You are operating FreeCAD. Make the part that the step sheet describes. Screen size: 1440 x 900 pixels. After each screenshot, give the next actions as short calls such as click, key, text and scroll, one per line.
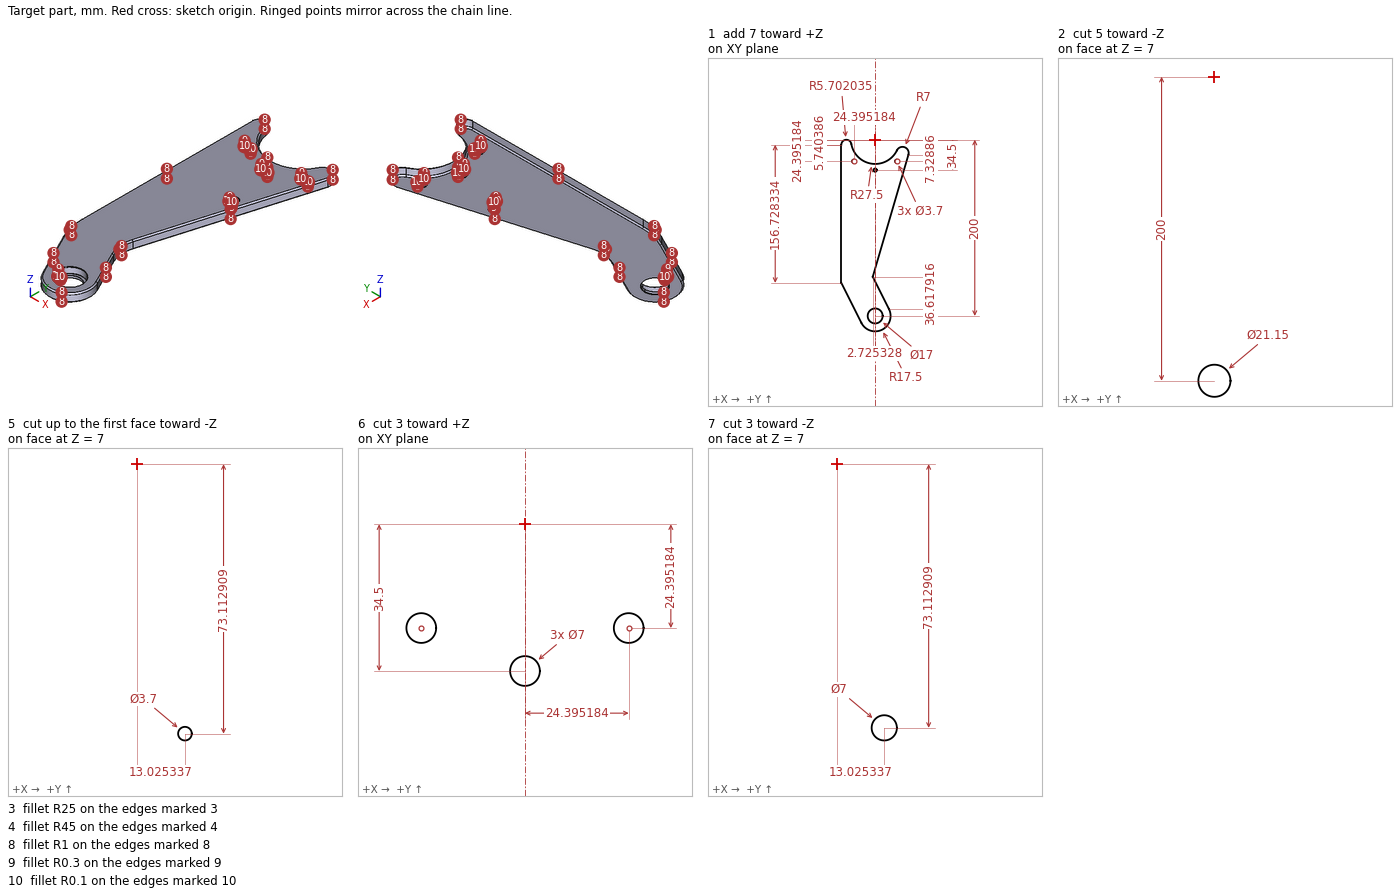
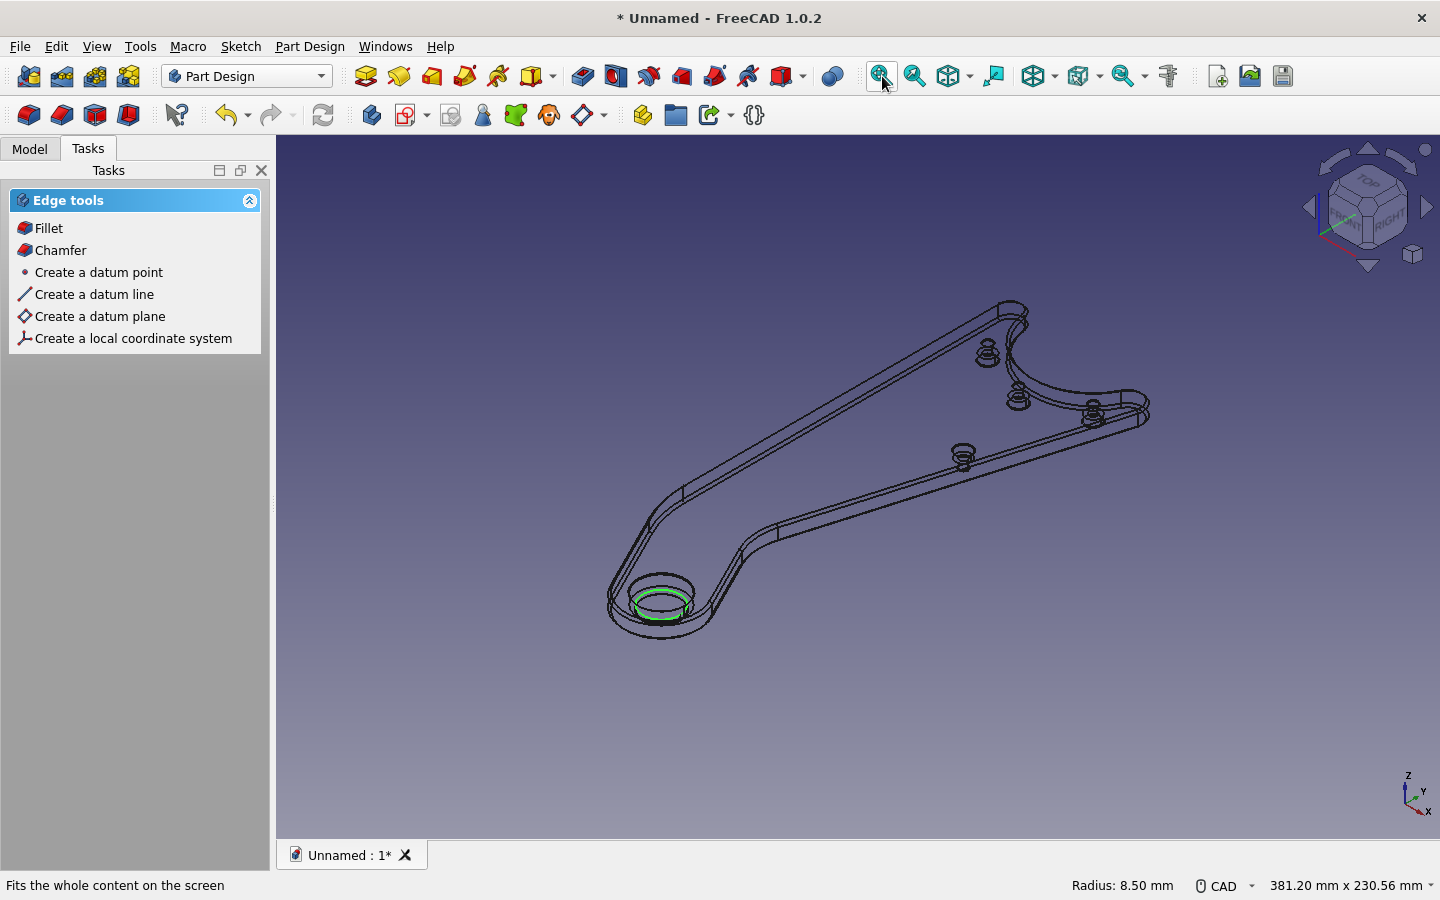
click(1008, 394, ctrl)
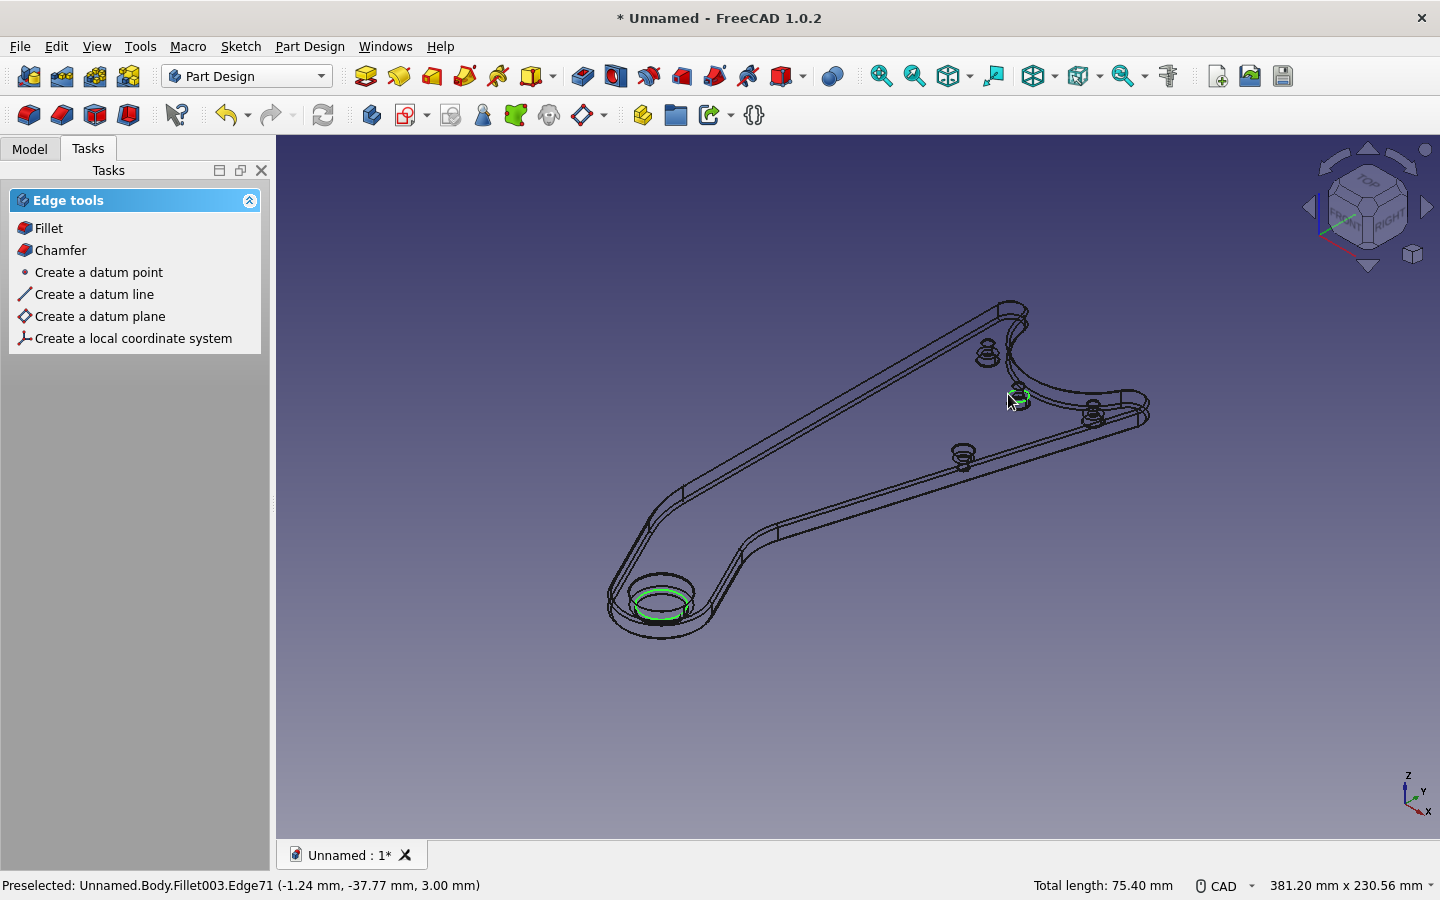
click(1083, 412, ctrl)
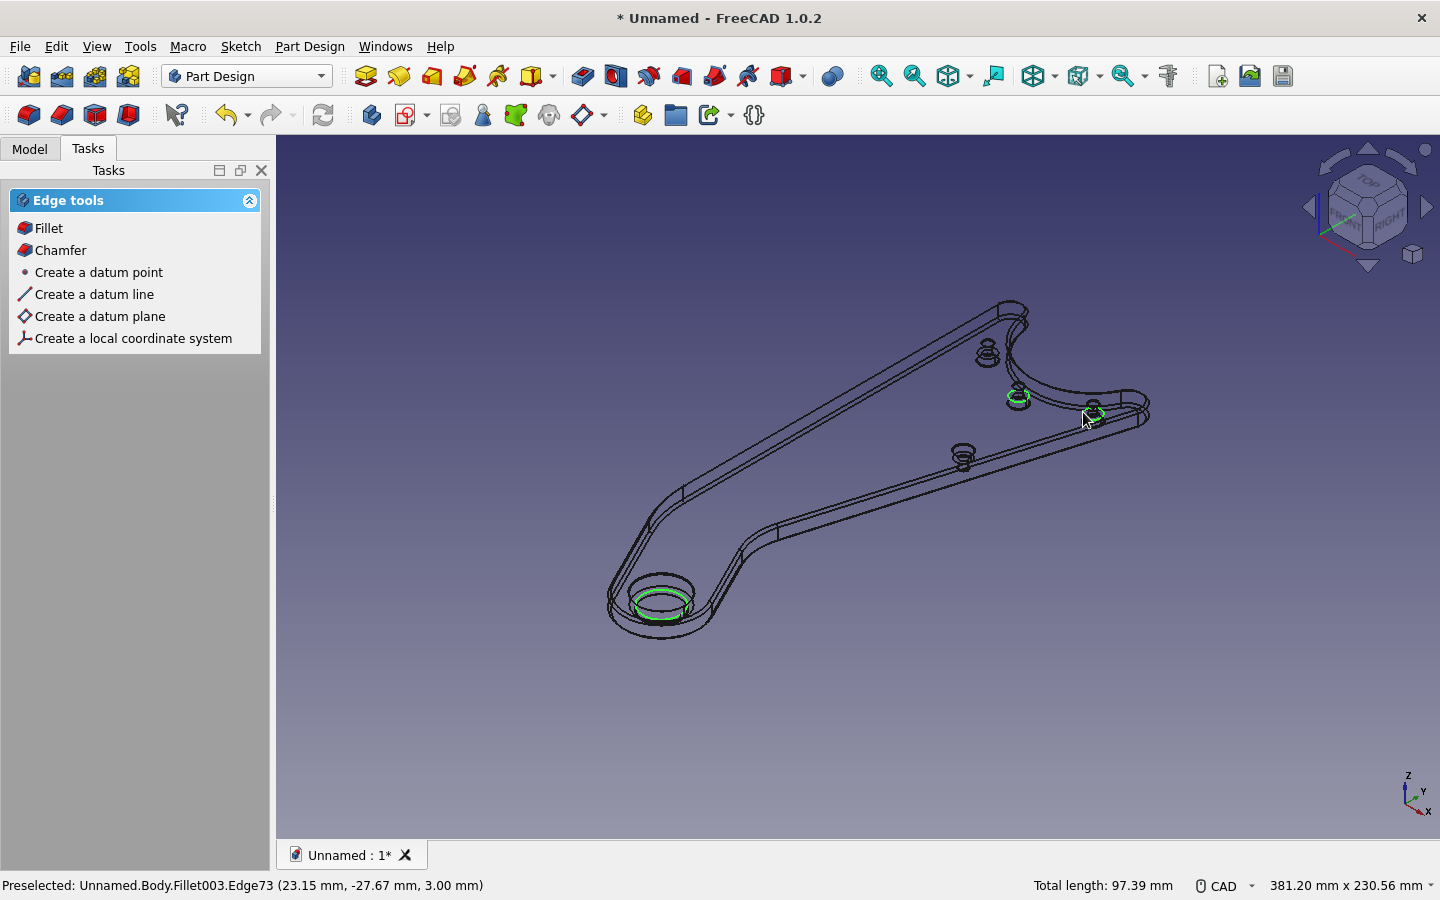
click(977, 351, ctrl)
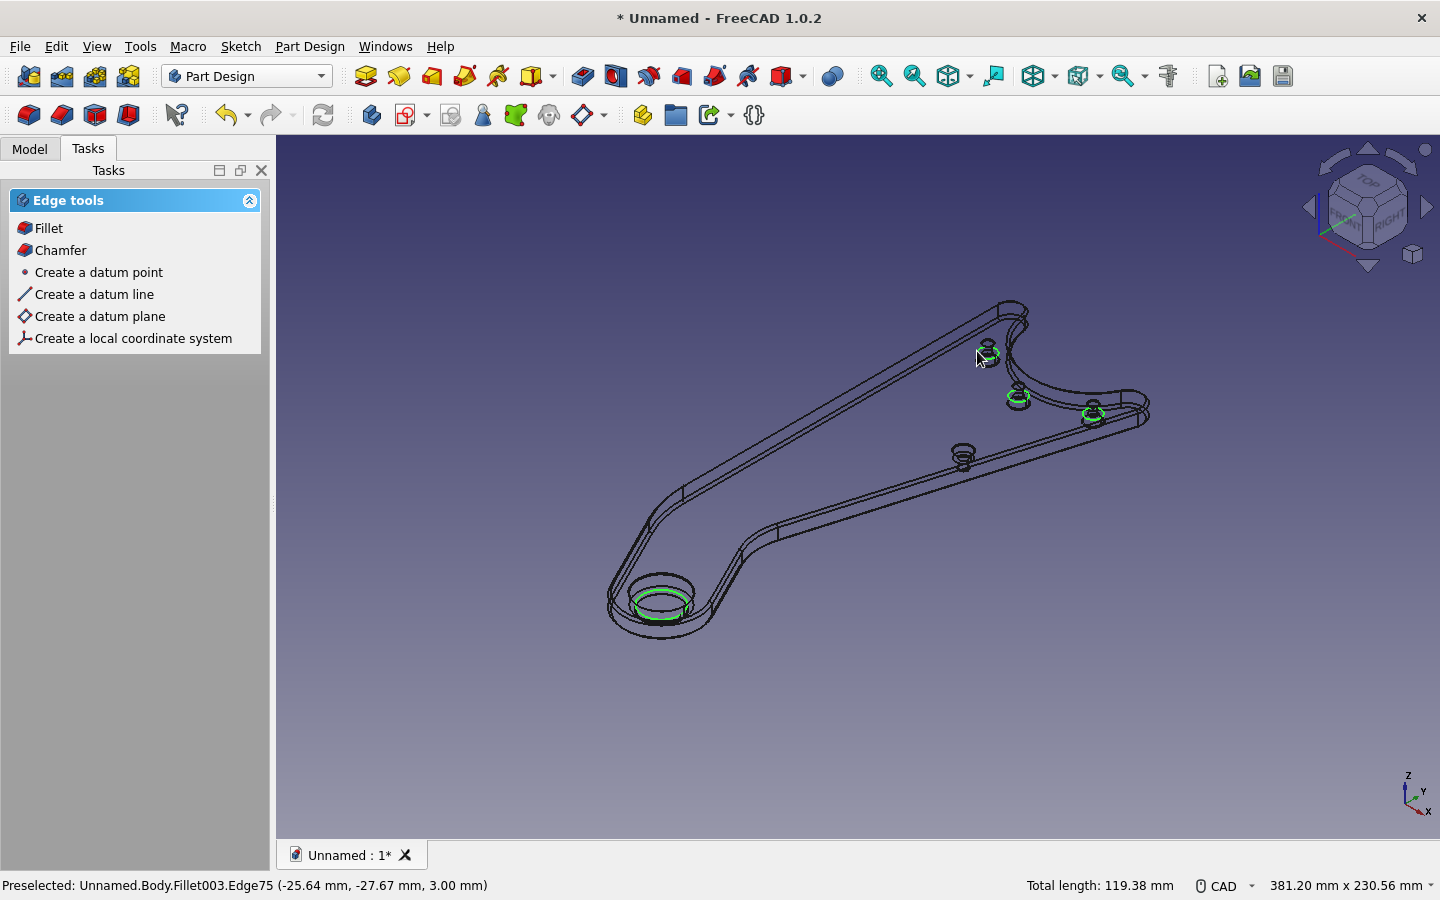
scroll(639, 591, up, 6)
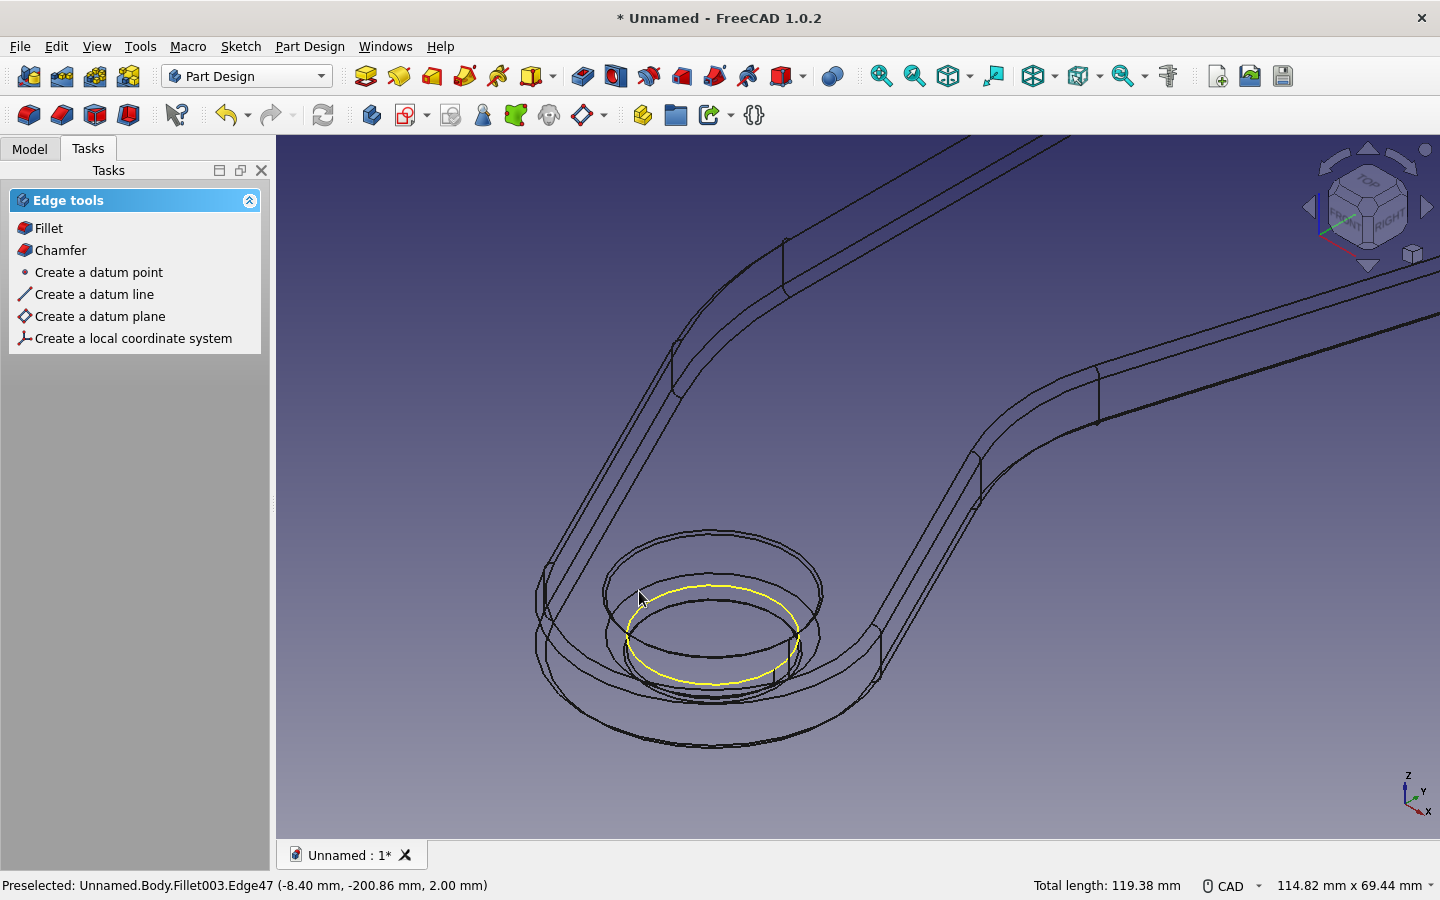
click(637, 590, ctrl)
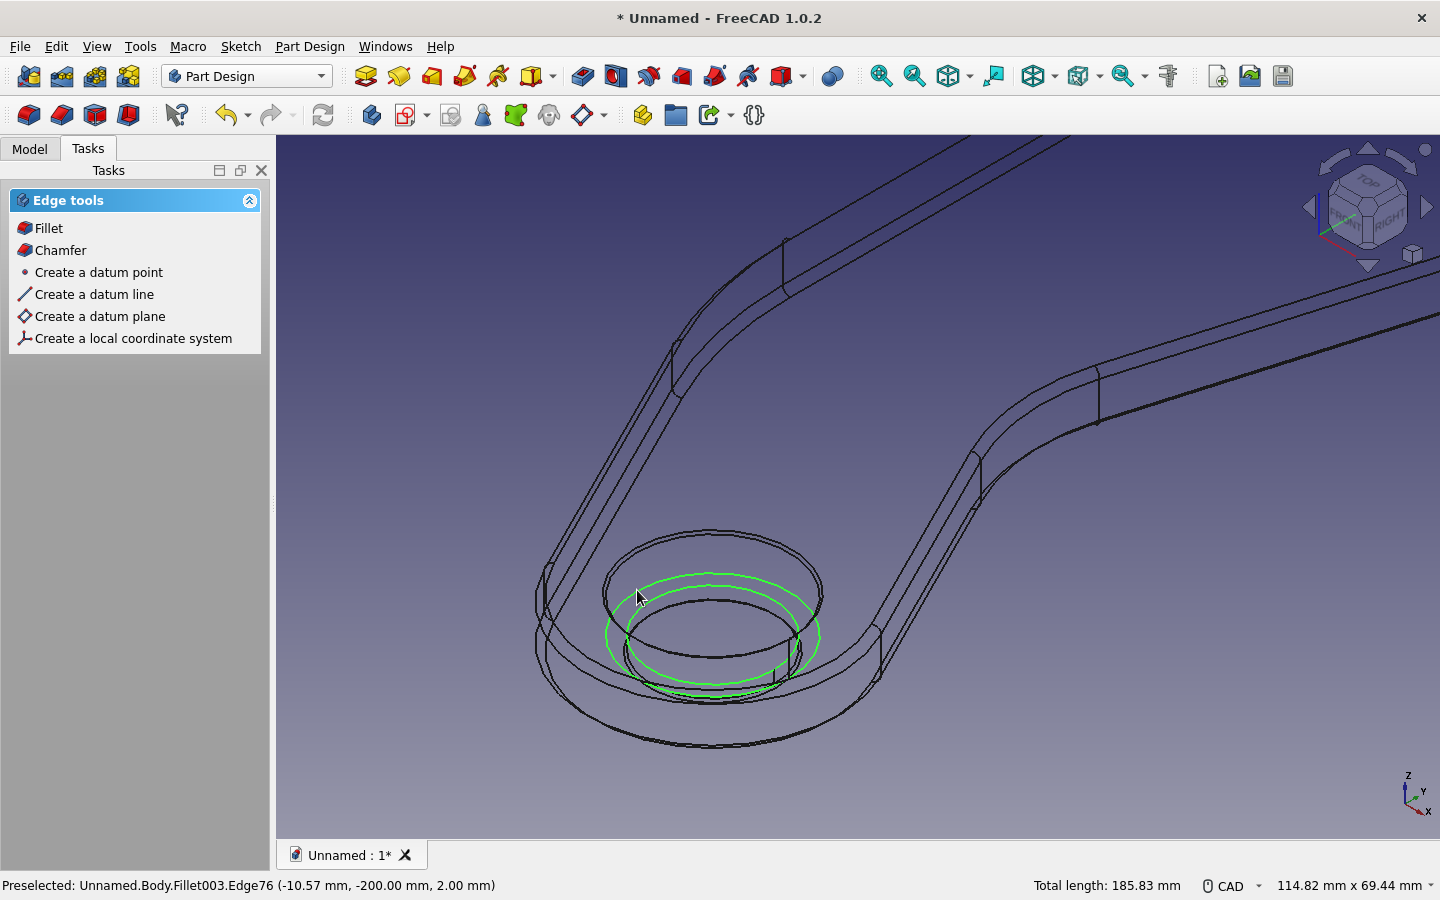
click(882, 76)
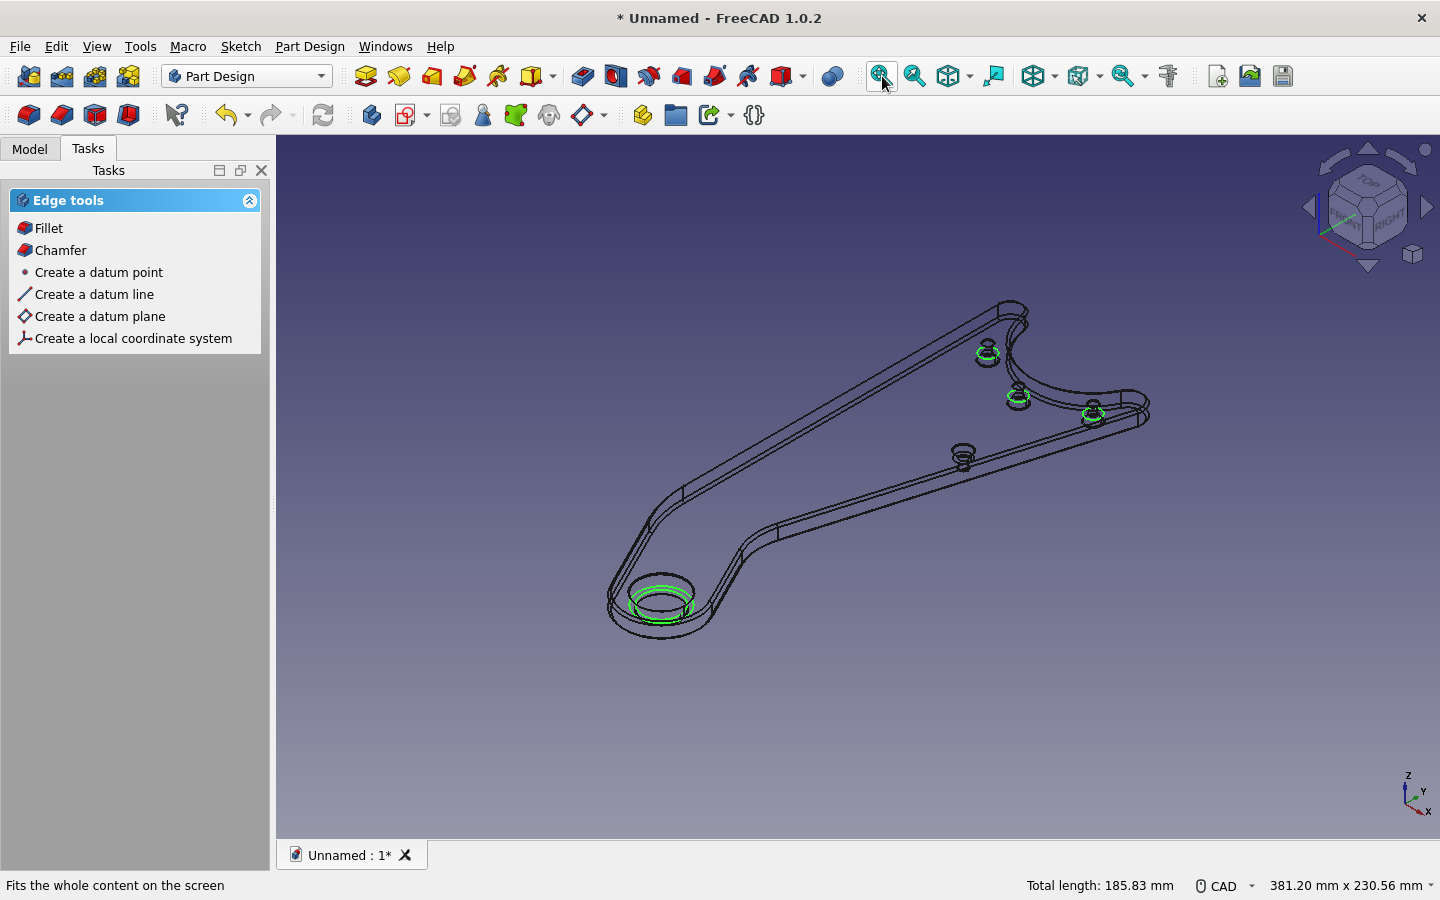
key(2)